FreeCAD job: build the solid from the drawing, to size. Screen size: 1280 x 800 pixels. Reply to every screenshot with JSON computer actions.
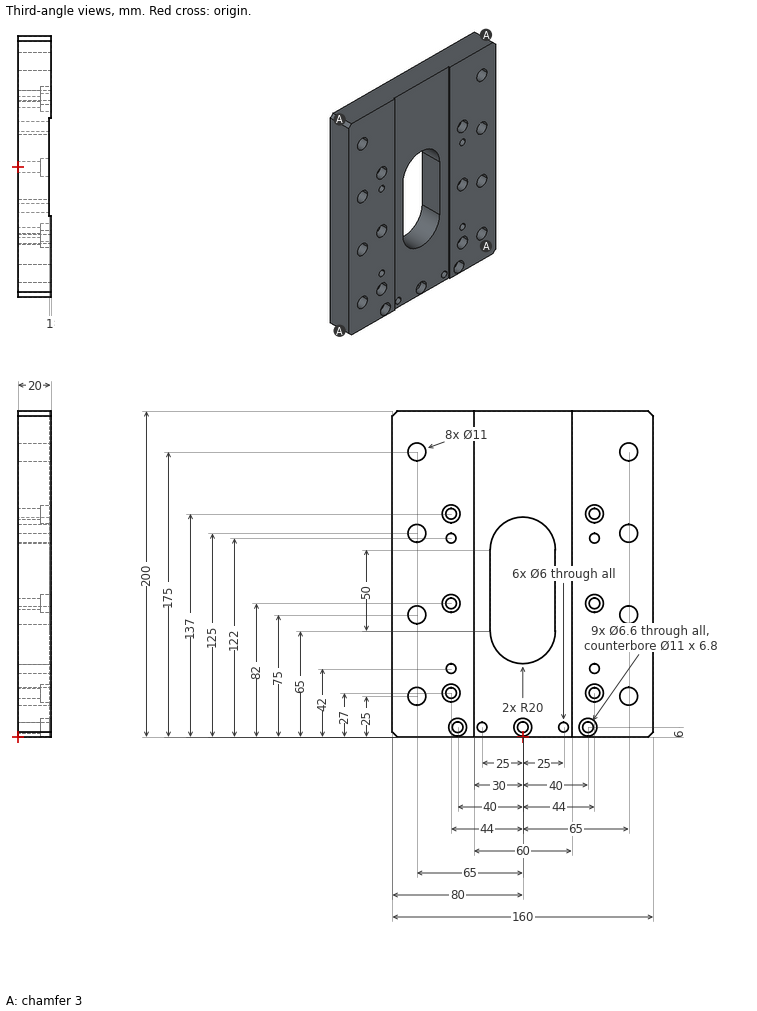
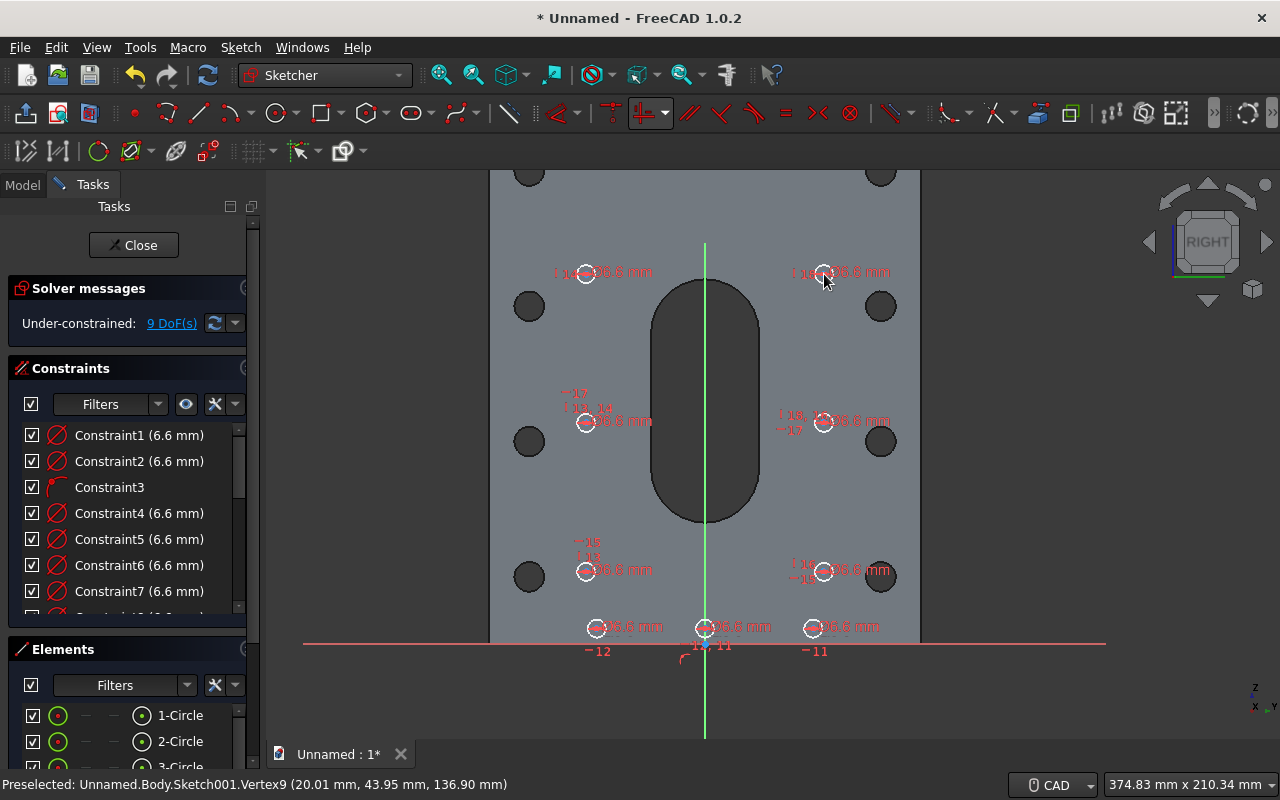
{"action": "left_click", "coordinate": [586, 274]}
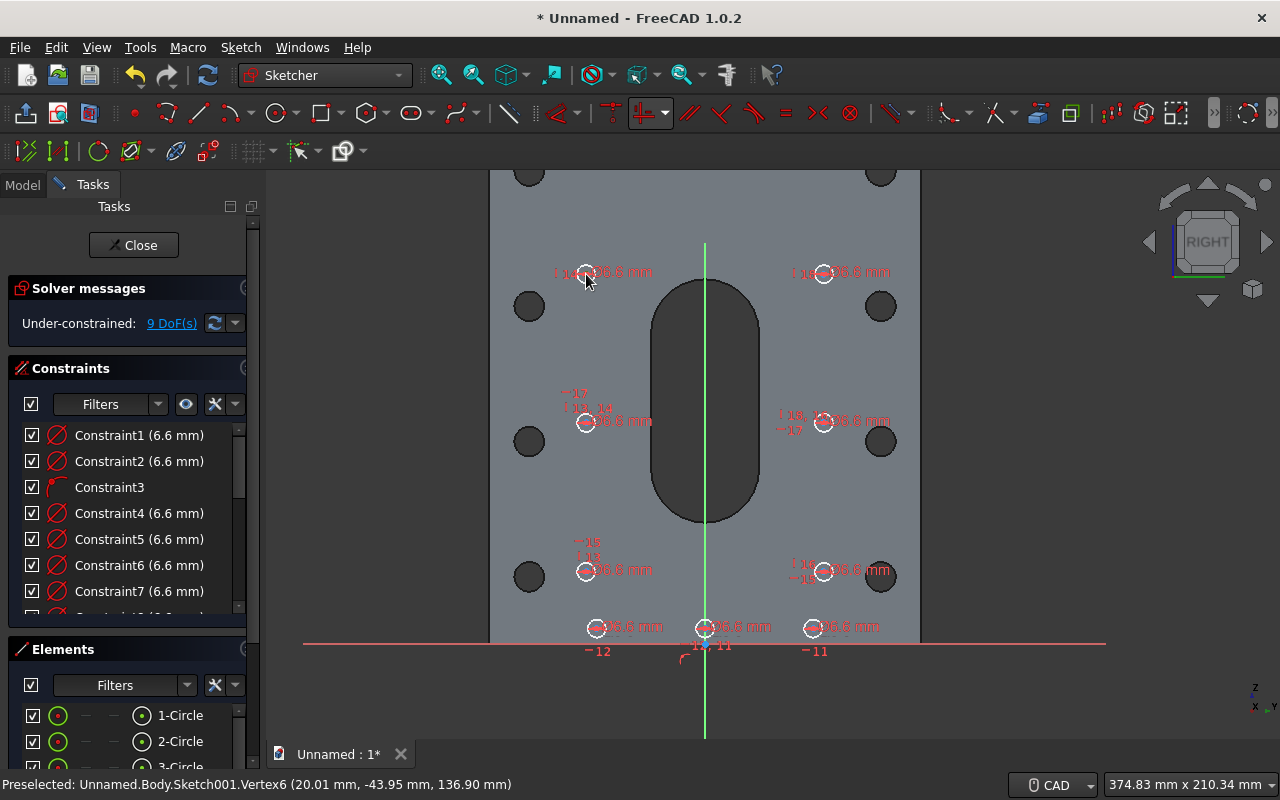
{"action": "left_click", "coordinate": [824, 274]}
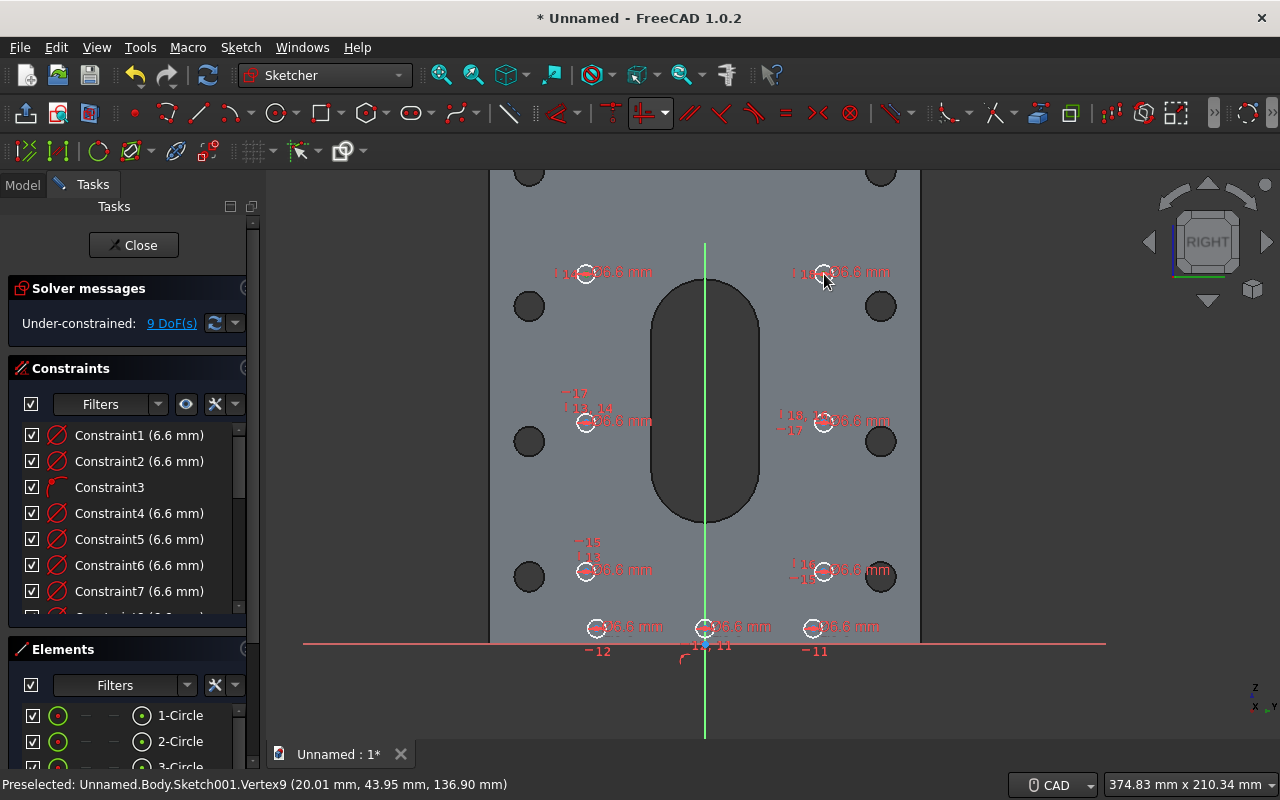
{"action": "key", "text": "h"}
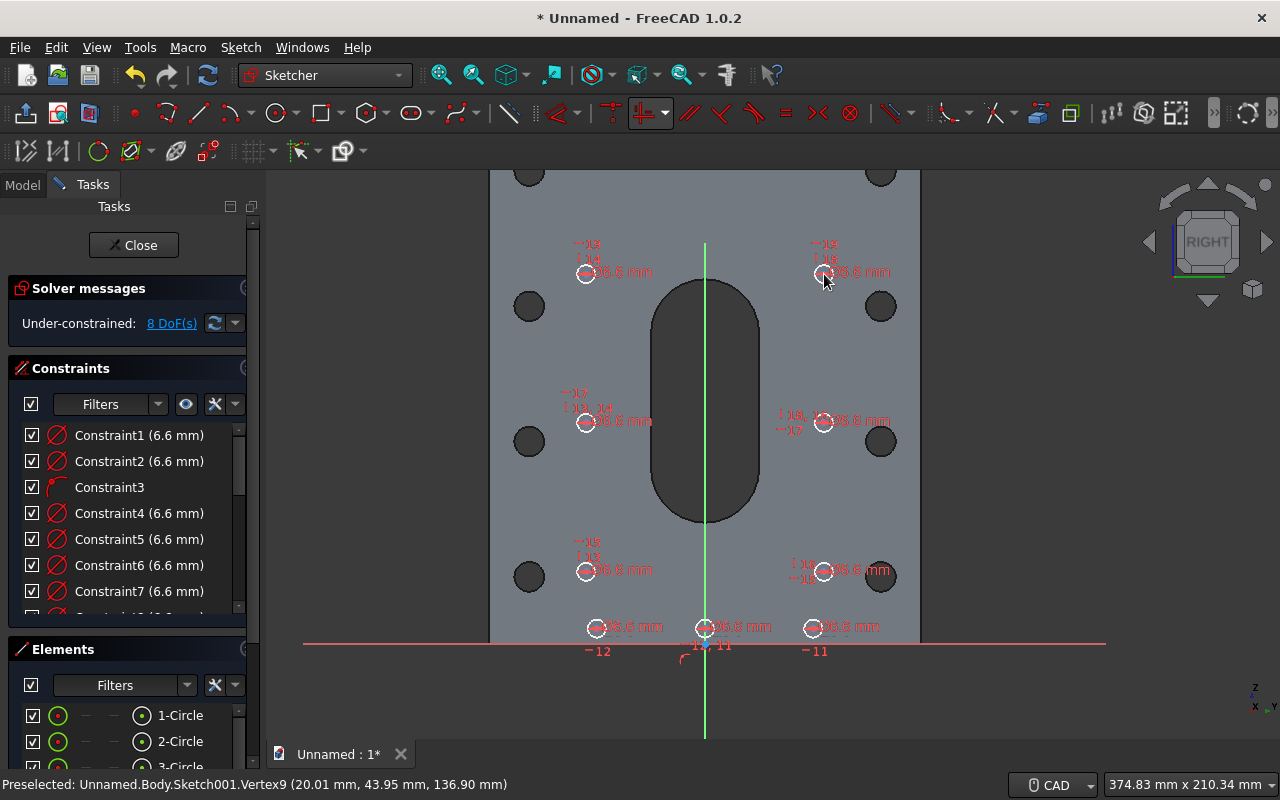
{"action": "key", "text": "d"}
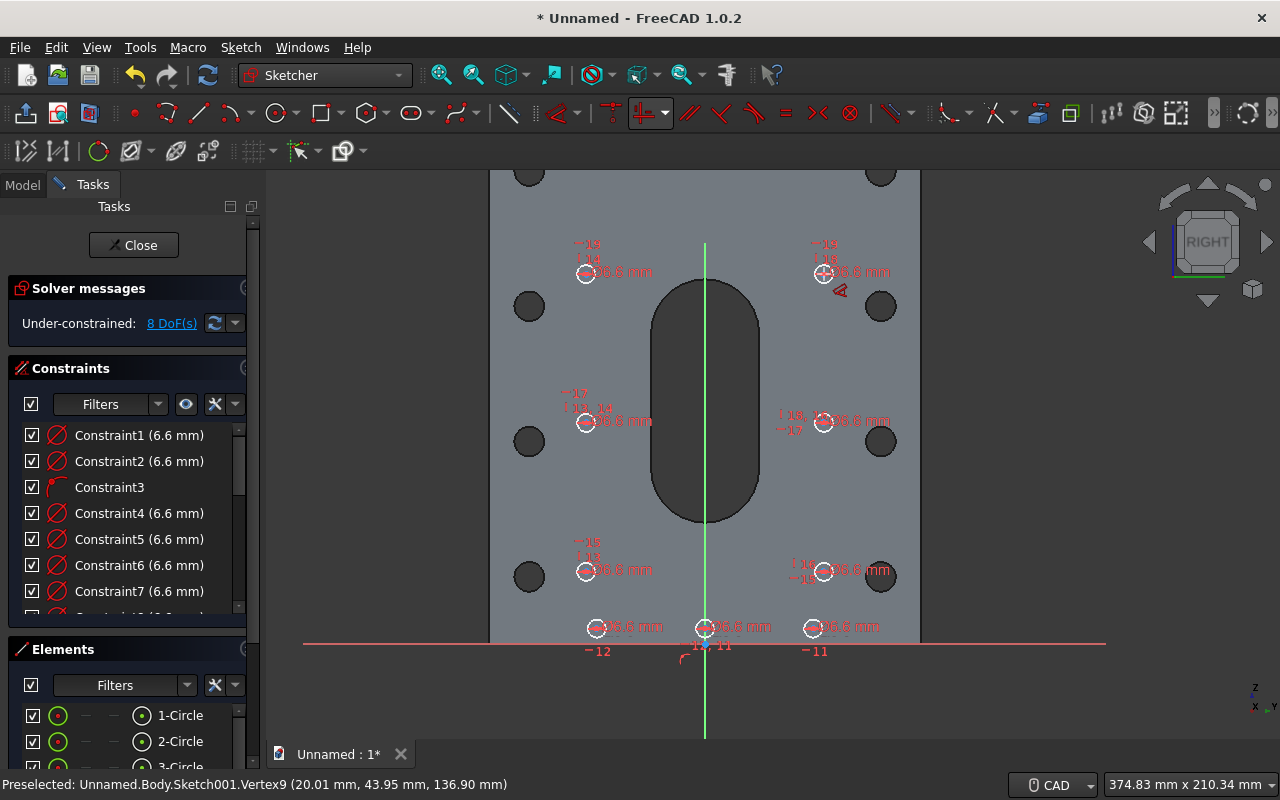
{"action": "scroll", "coordinate": [813, 629], "scroll_direction": "up", "scroll_amount": 5}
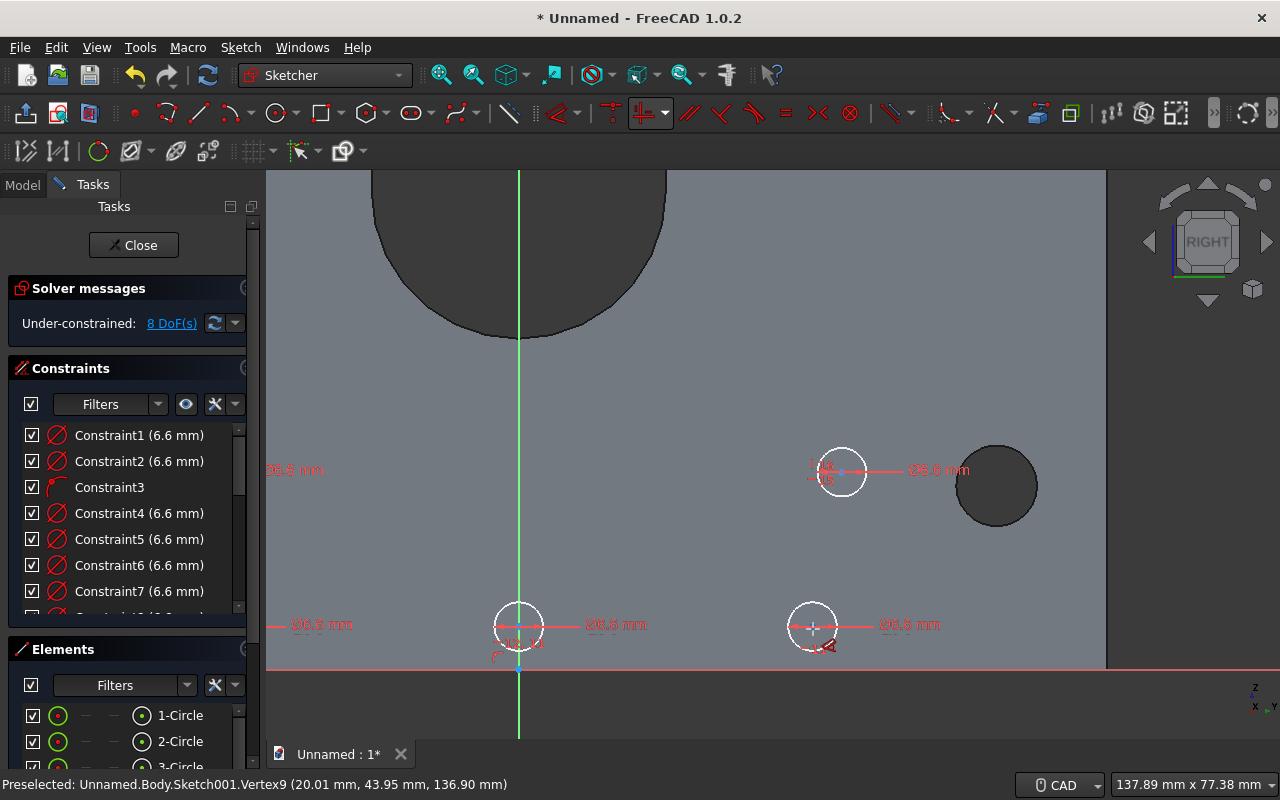
{"action": "left_click", "coordinate": [813, 627]}
{"action": "left_click", "coordinate": [847, 648]}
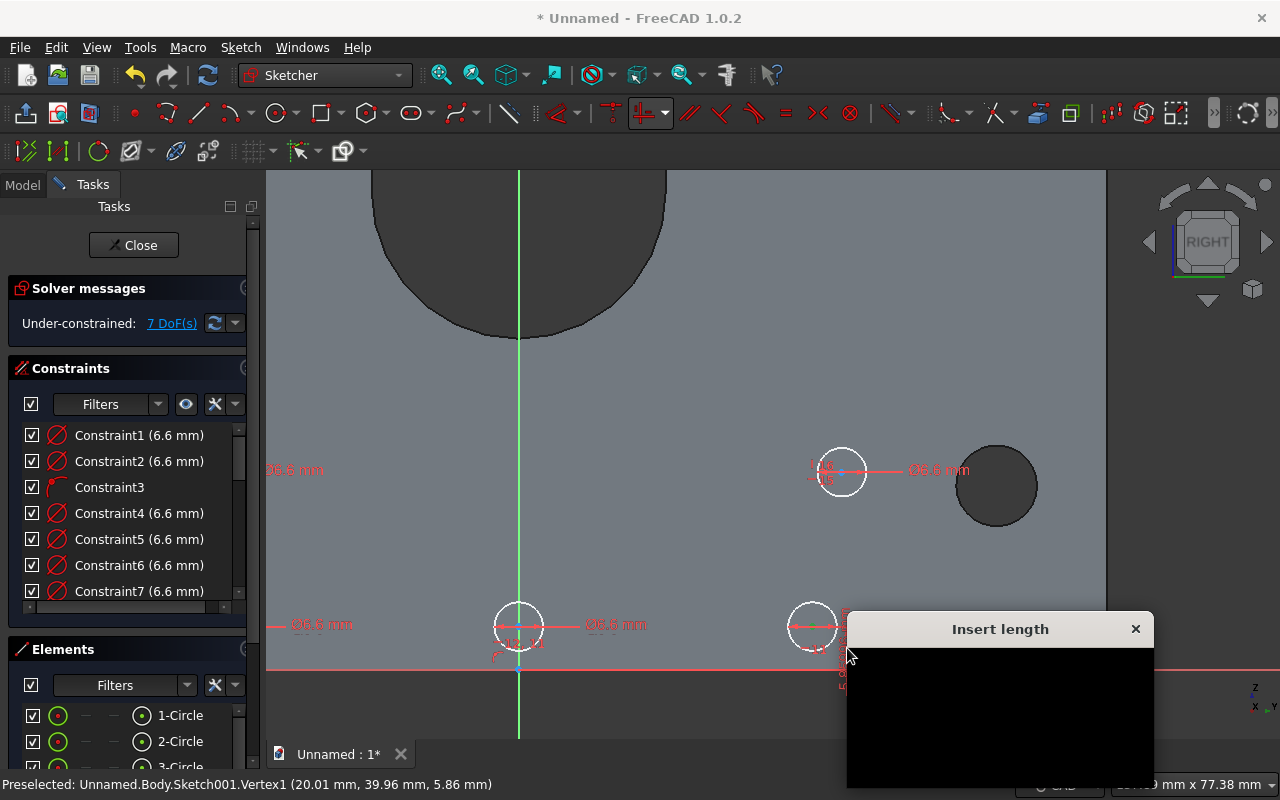
{"action": "type", "text": "6"}
{"action": "key", "text": "Return"}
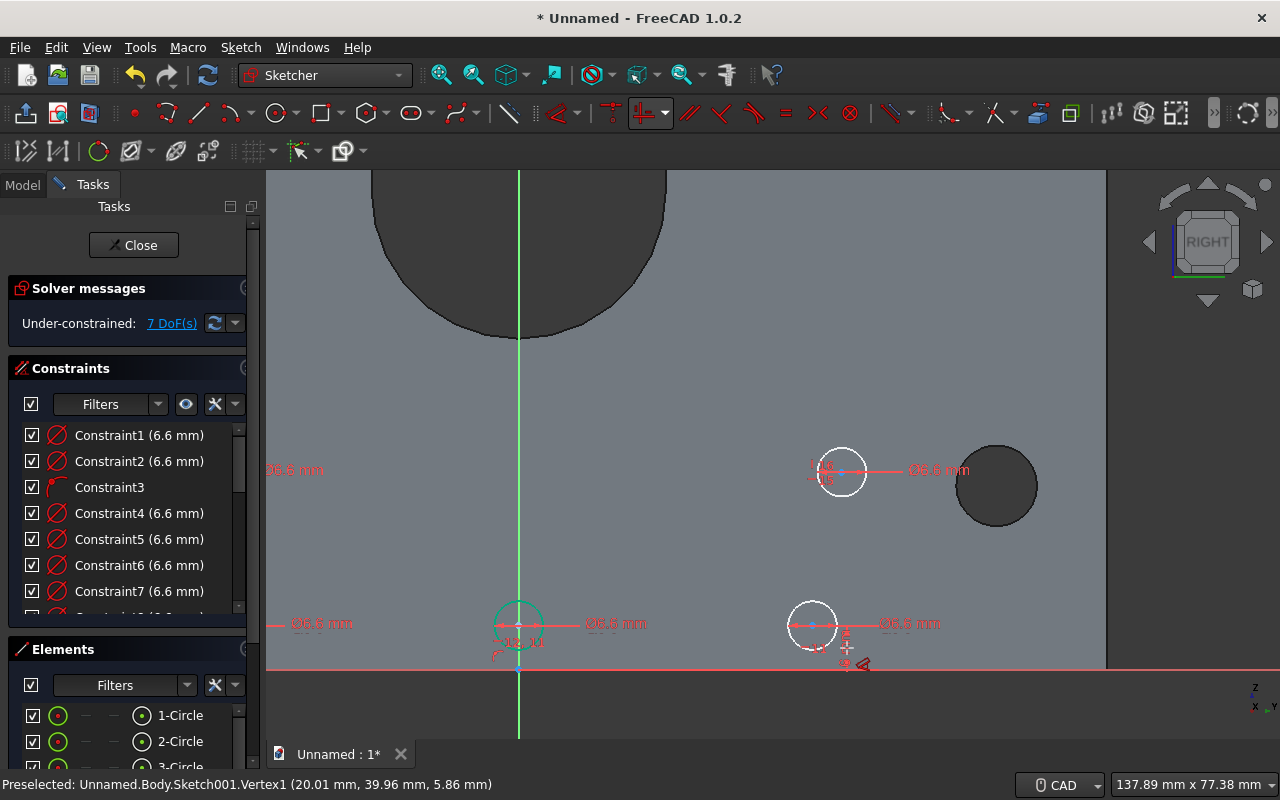
{"action": "left_click", "coordinate": [813, 626]}
{"action": "left_click", "coordinate": [666, 704]}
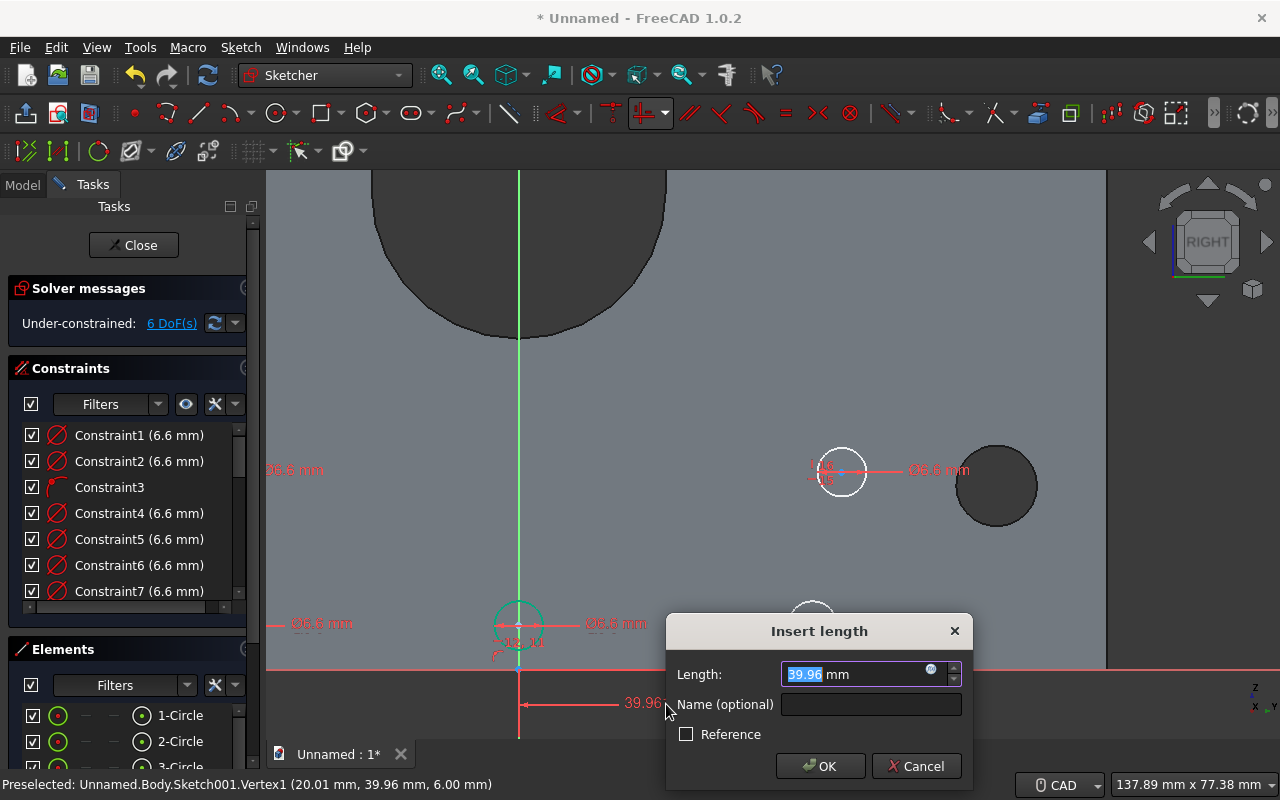
{"action": "type", "text": "40"}
{"action": "key", "text": "Return"}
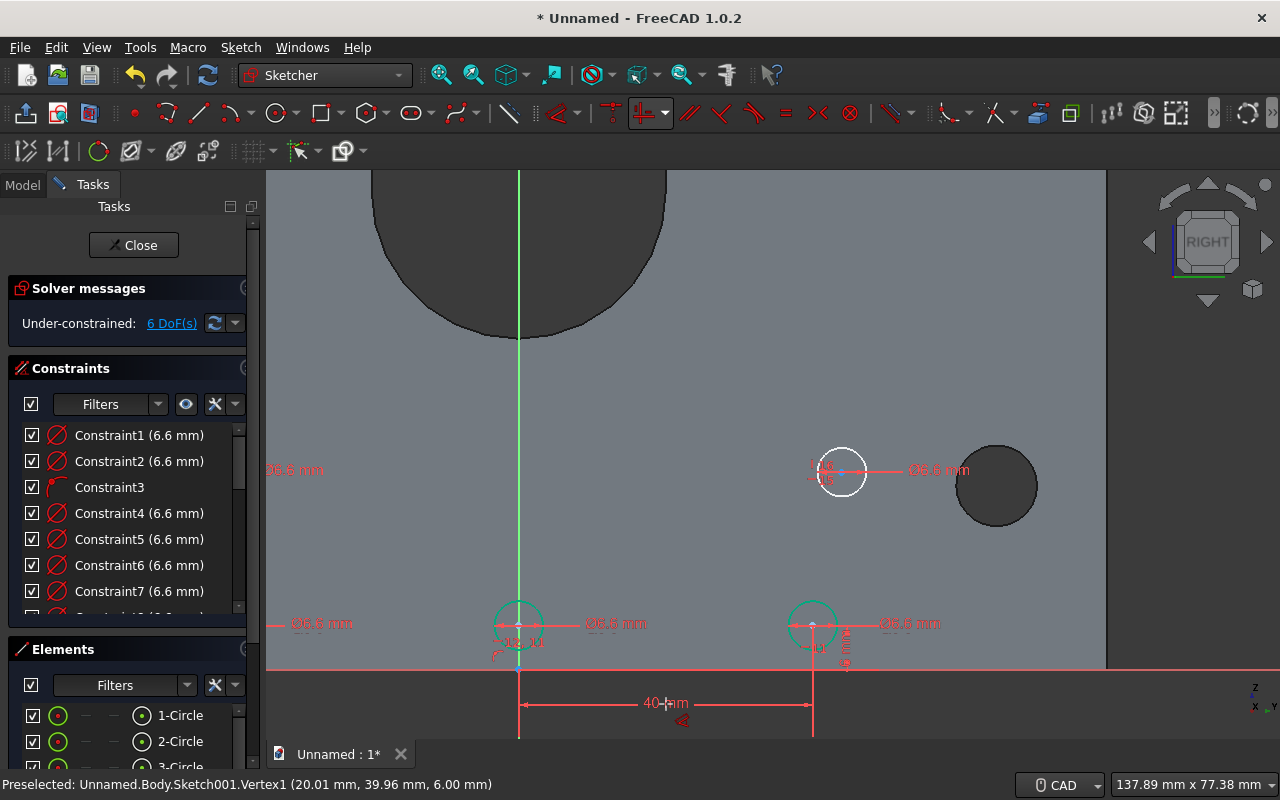
{"action": "scroll", "coordinate": [813, 629], "scroll_direction": "down", "scroll_amount": 5}